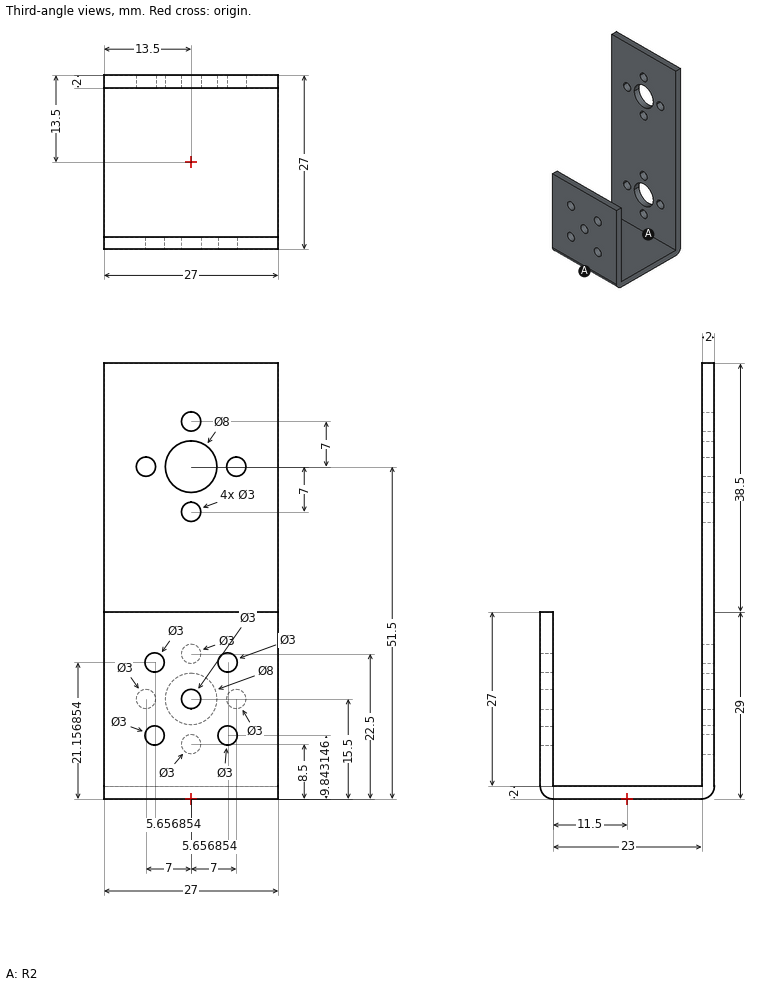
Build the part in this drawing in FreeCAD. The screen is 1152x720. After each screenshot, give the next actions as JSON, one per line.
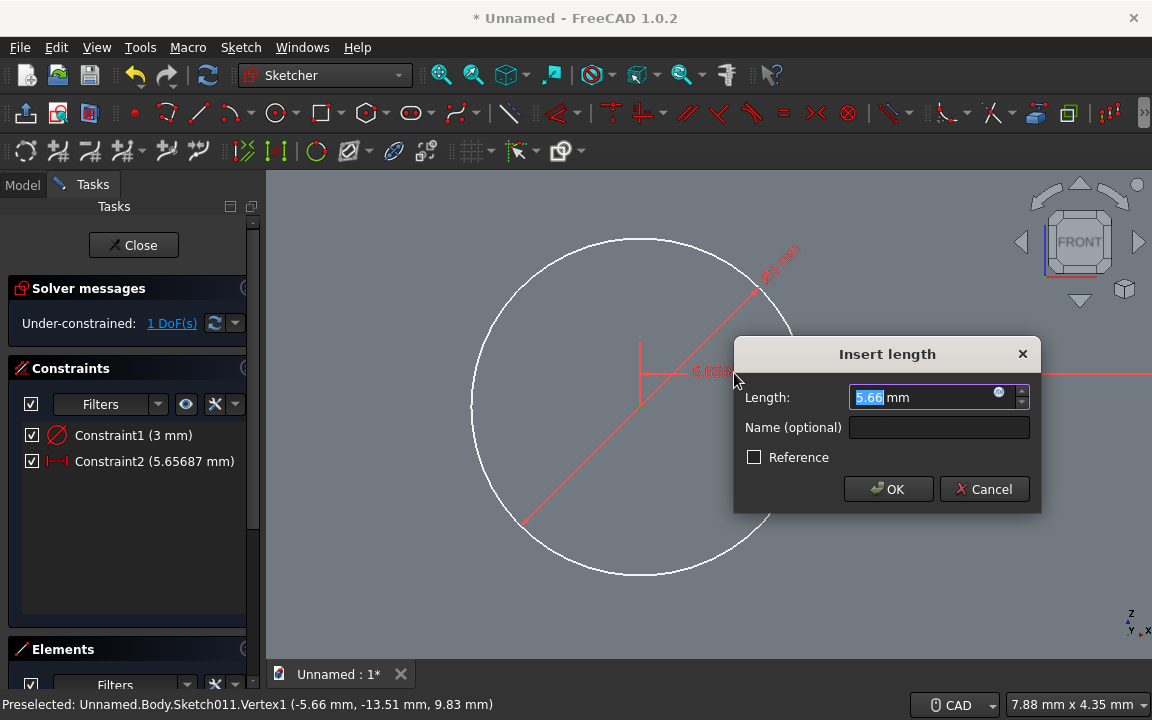
{"action": "type", "text": "5.656854"}
{"action": "key", "text": "Return"}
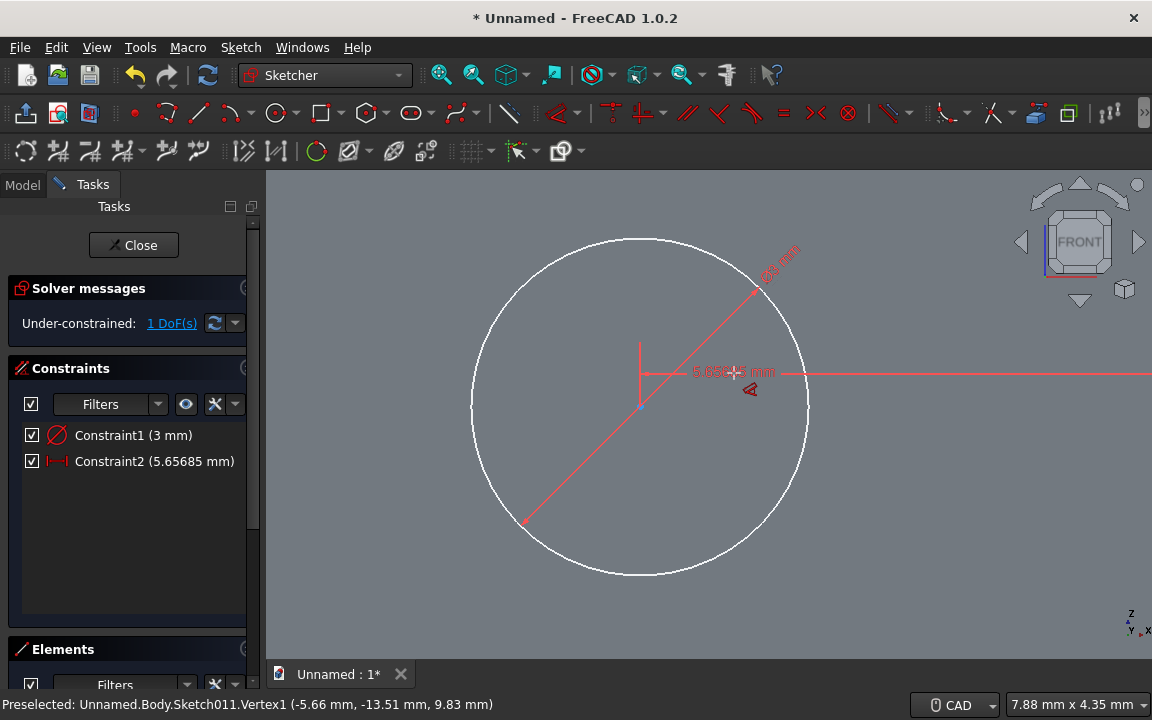
{"action": "left_click", "coordinate": [640, 407]}
{"action": "left_click", "coordinate": [606, 519]}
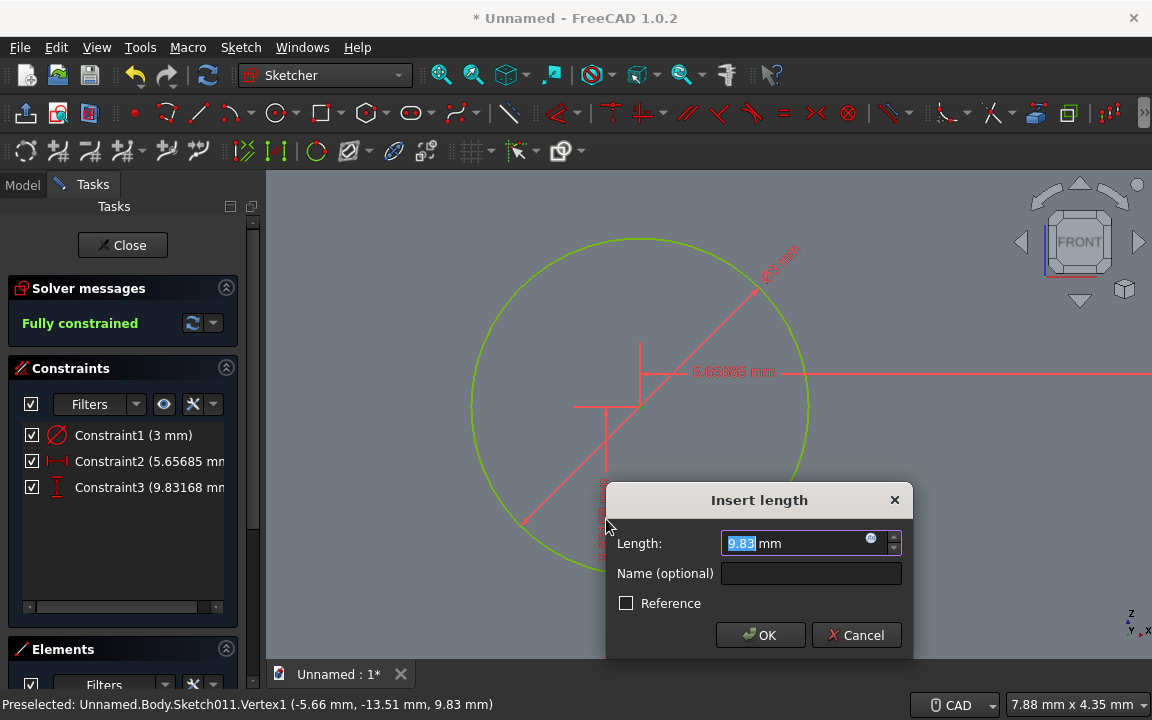
{"action": "type", "text": "9.843146"}
{"action": "key", "text": "Return"}
{"action": "key", "text": "Escape"}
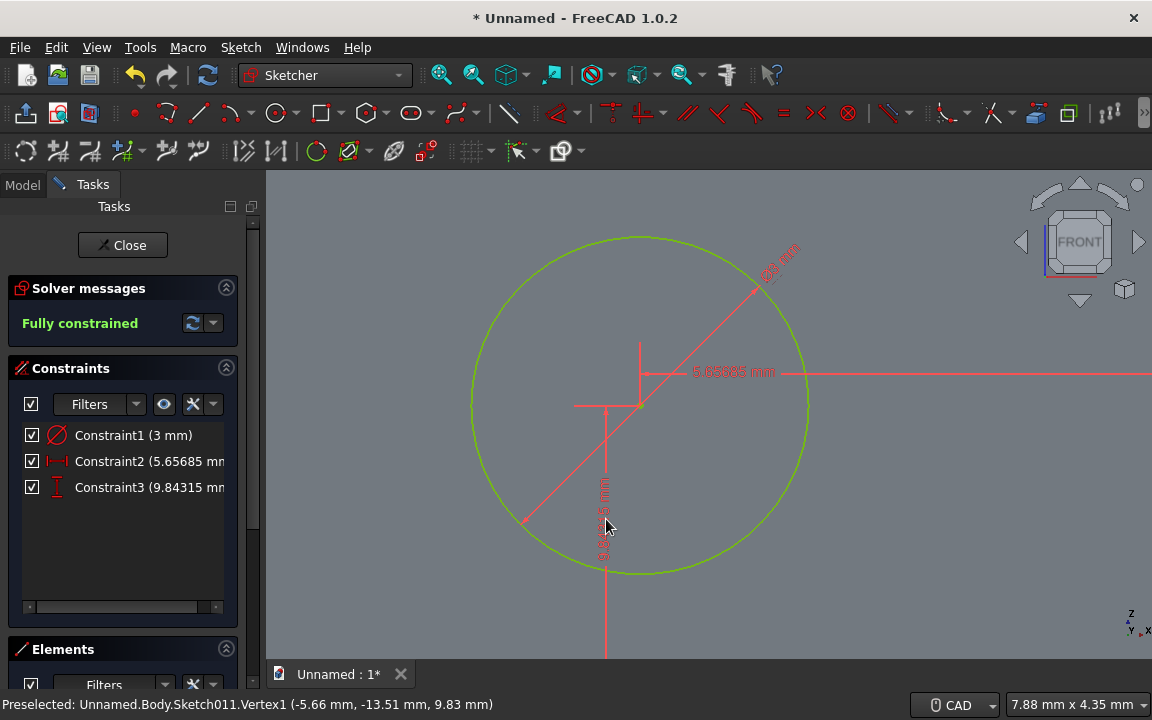
{"action": "left_click", "coordinate": [123, 245]}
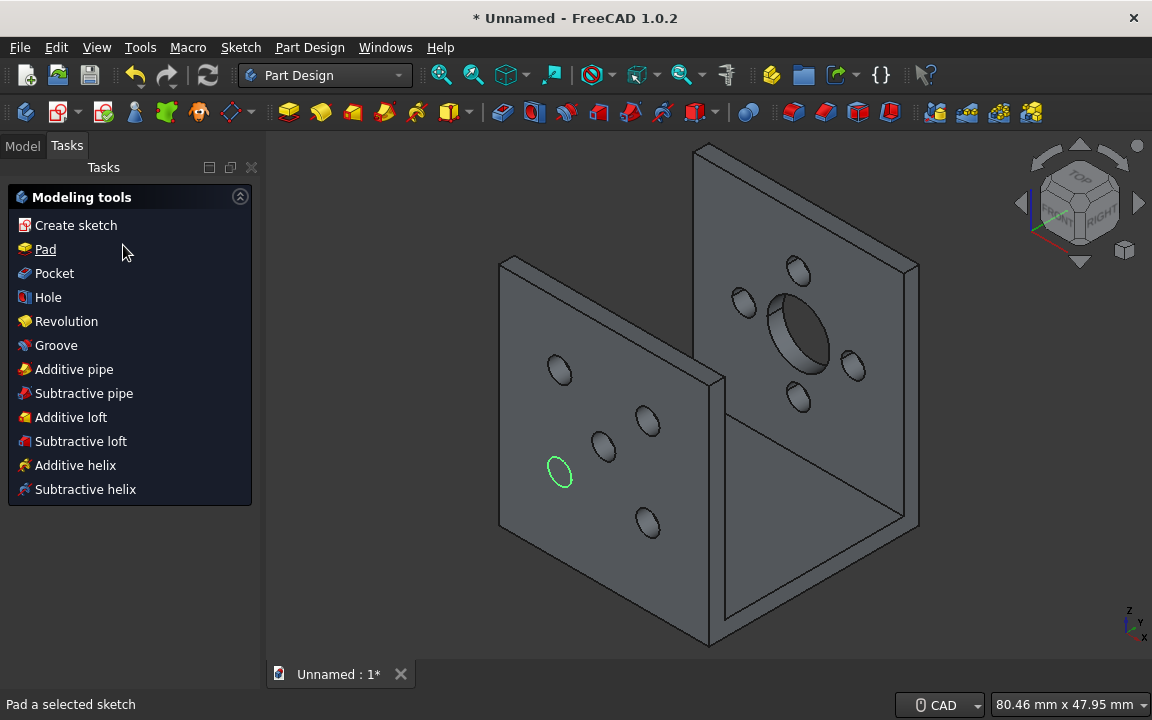
{"action": "left_click", "coordinate": [504, 112]}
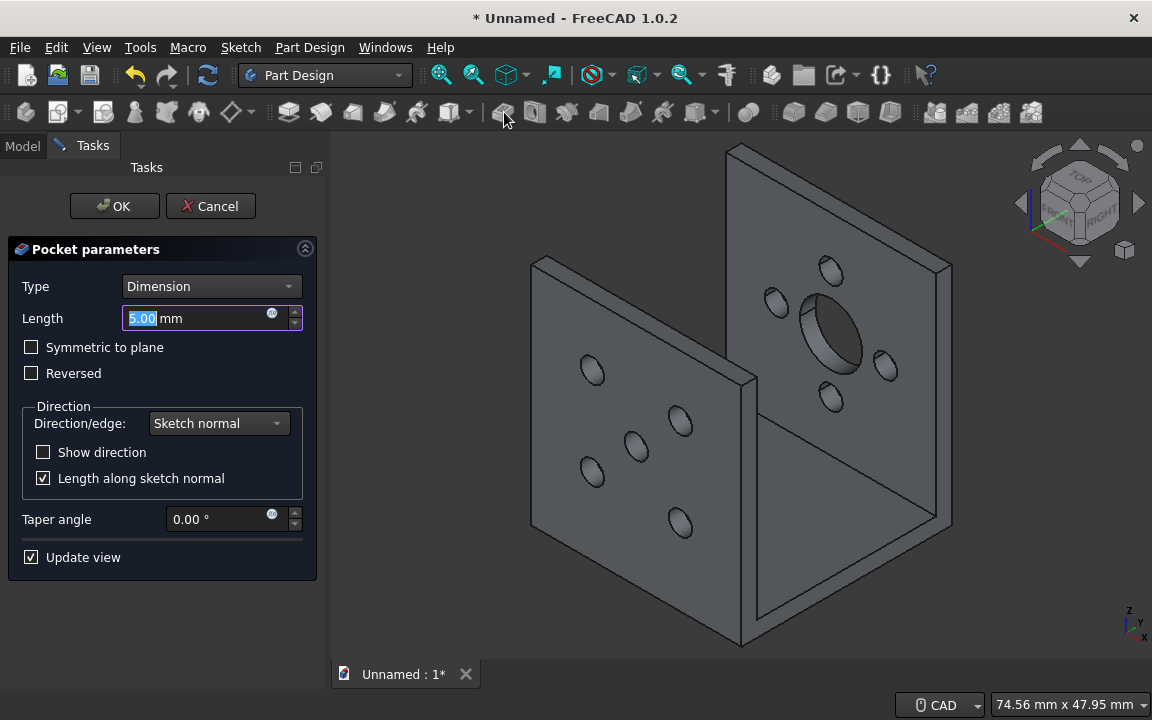
{"action": "left_click", "coordinate": [212, 286]}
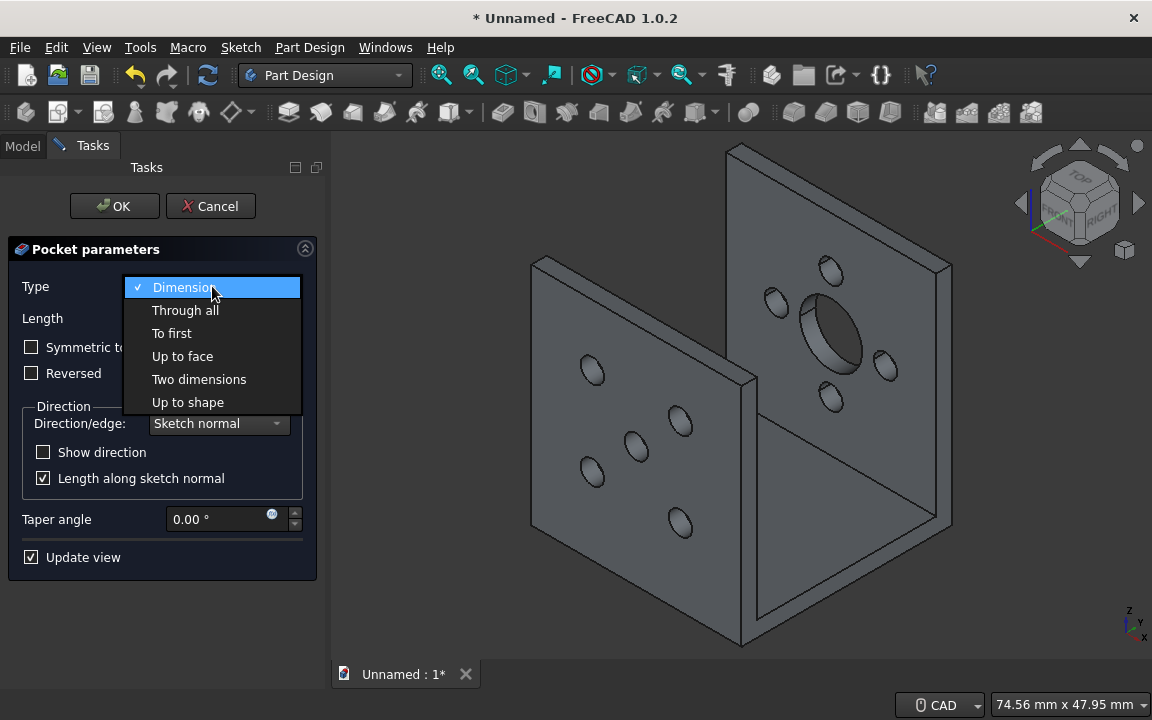
{"action": "left_click", "coordinate": [212, 334]}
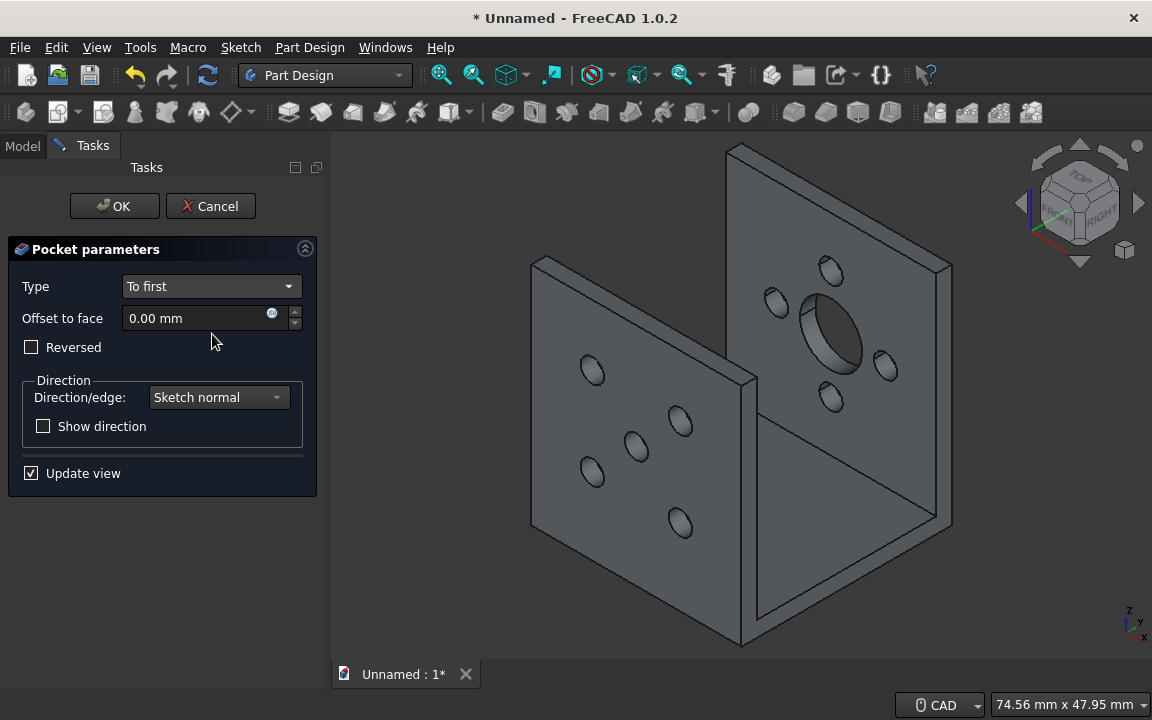
{"action": "left_click", "coordinate": [115, 206]}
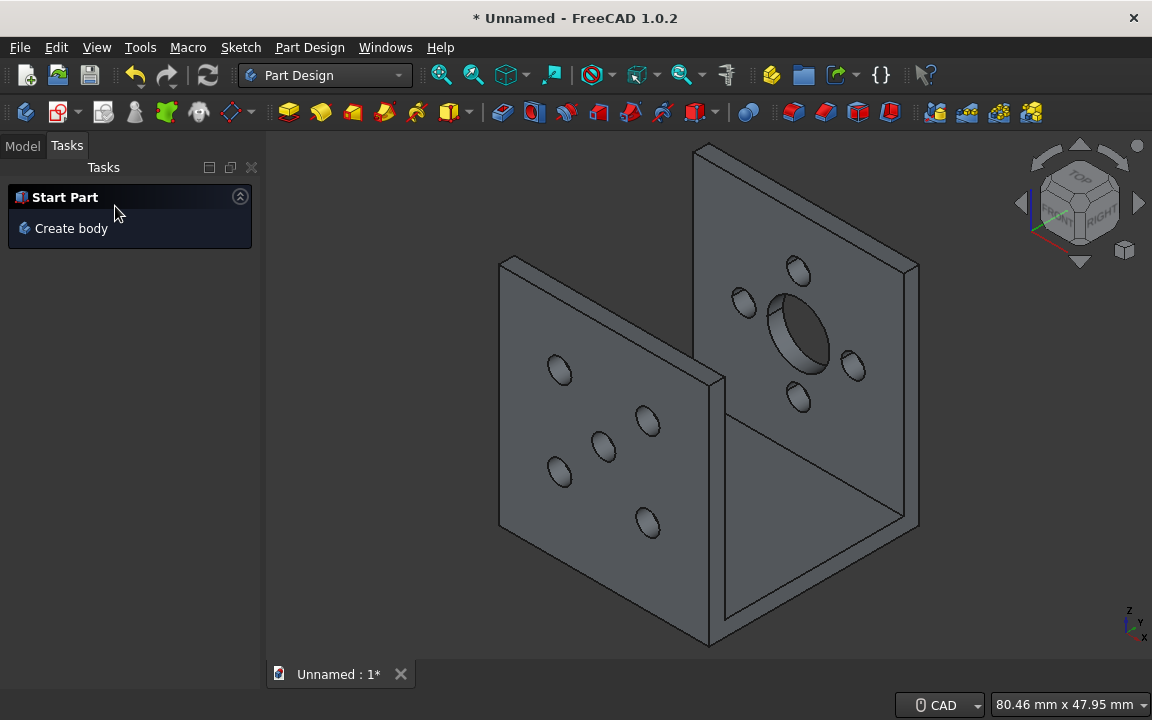
{"action": "key", "text": "2"}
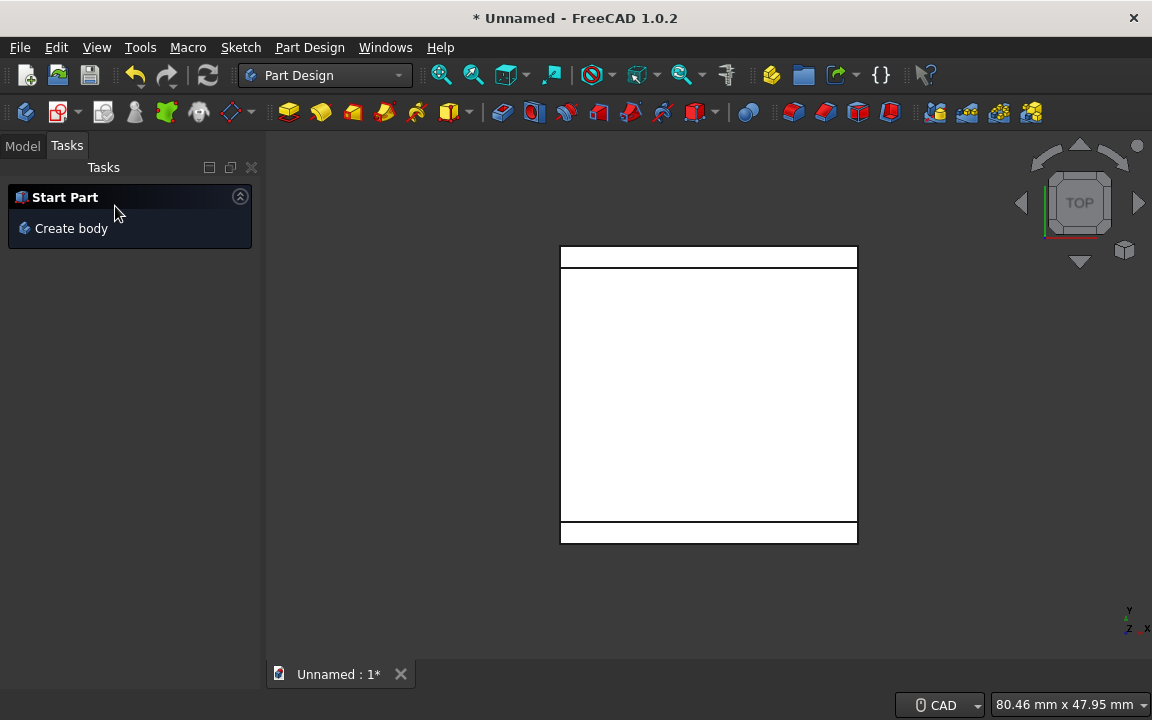
{"action": "key", "text": "0"}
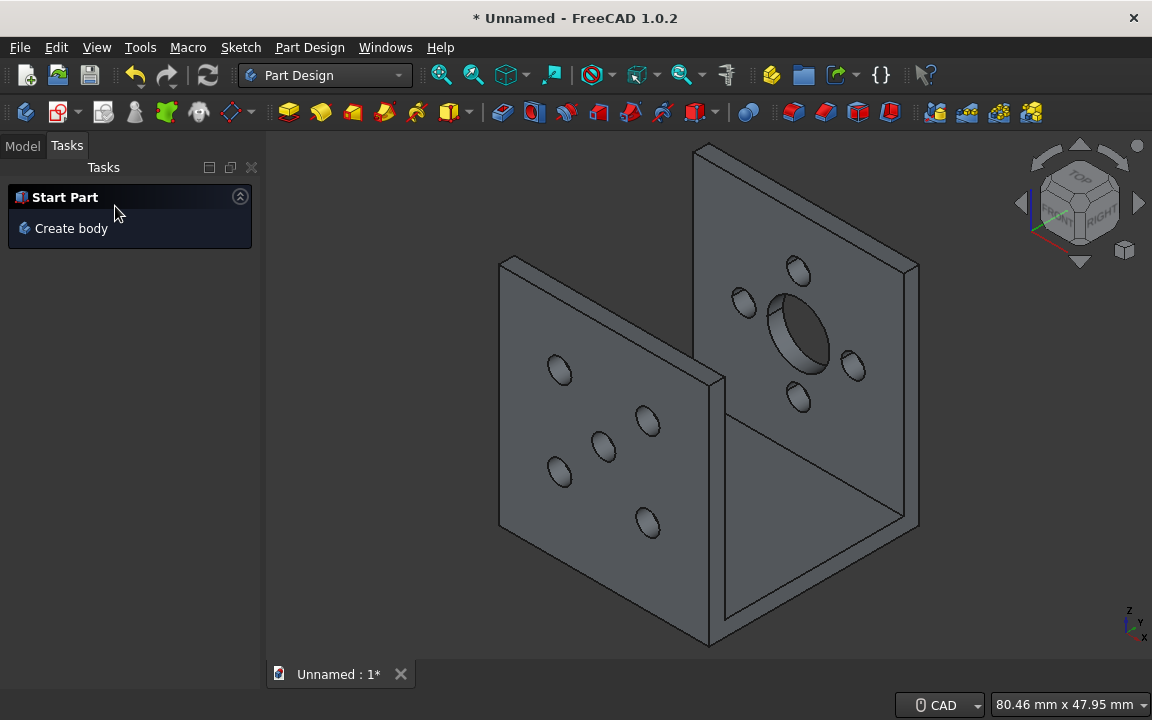
{"action": "key", "text": "1"}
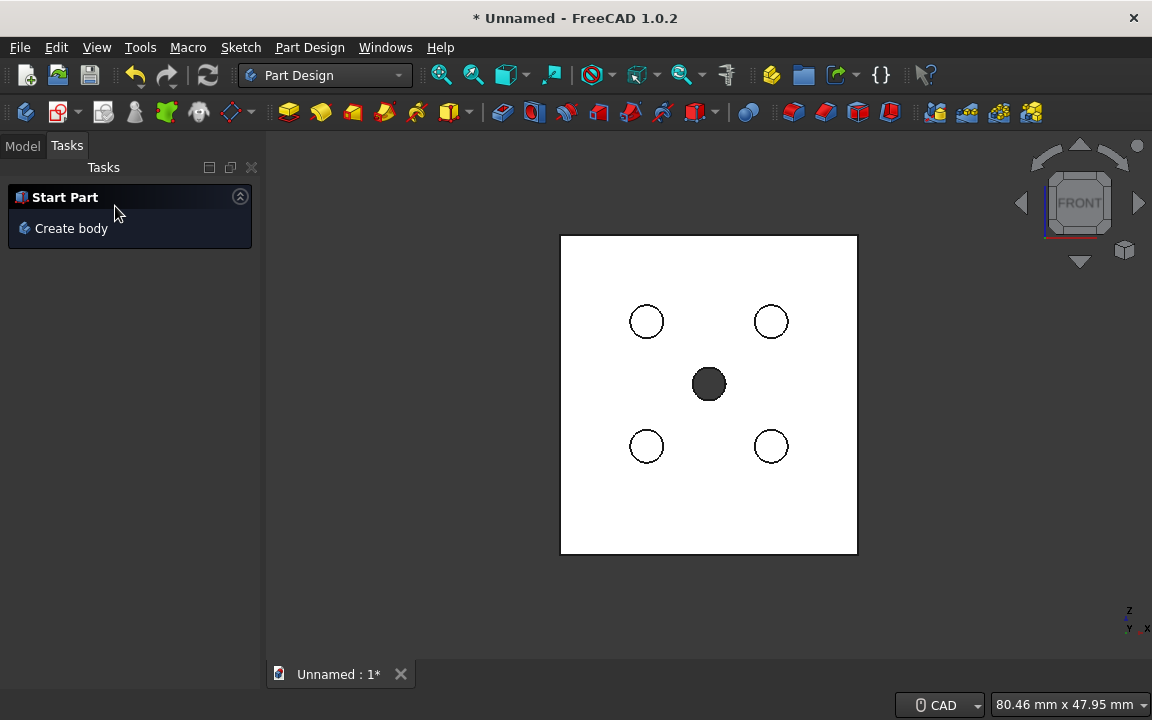
{"action": "left_click", "coordinate": [709, 554]}